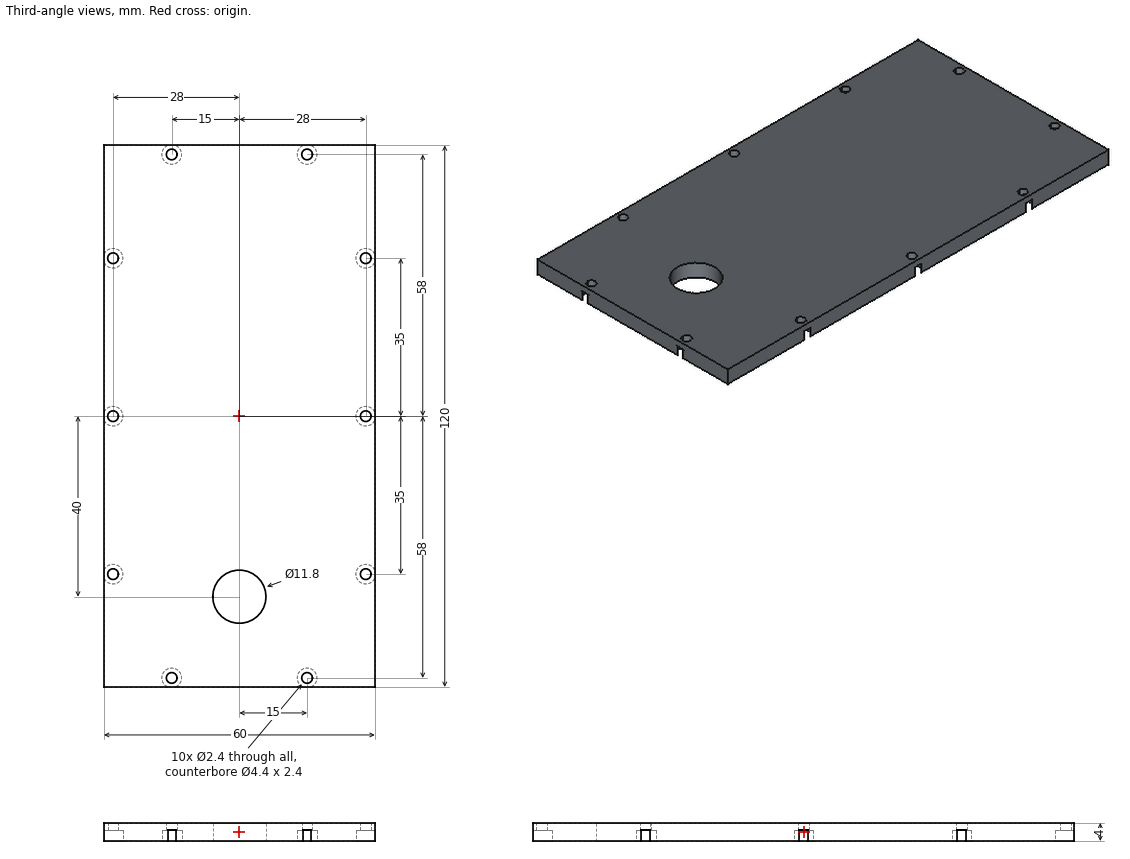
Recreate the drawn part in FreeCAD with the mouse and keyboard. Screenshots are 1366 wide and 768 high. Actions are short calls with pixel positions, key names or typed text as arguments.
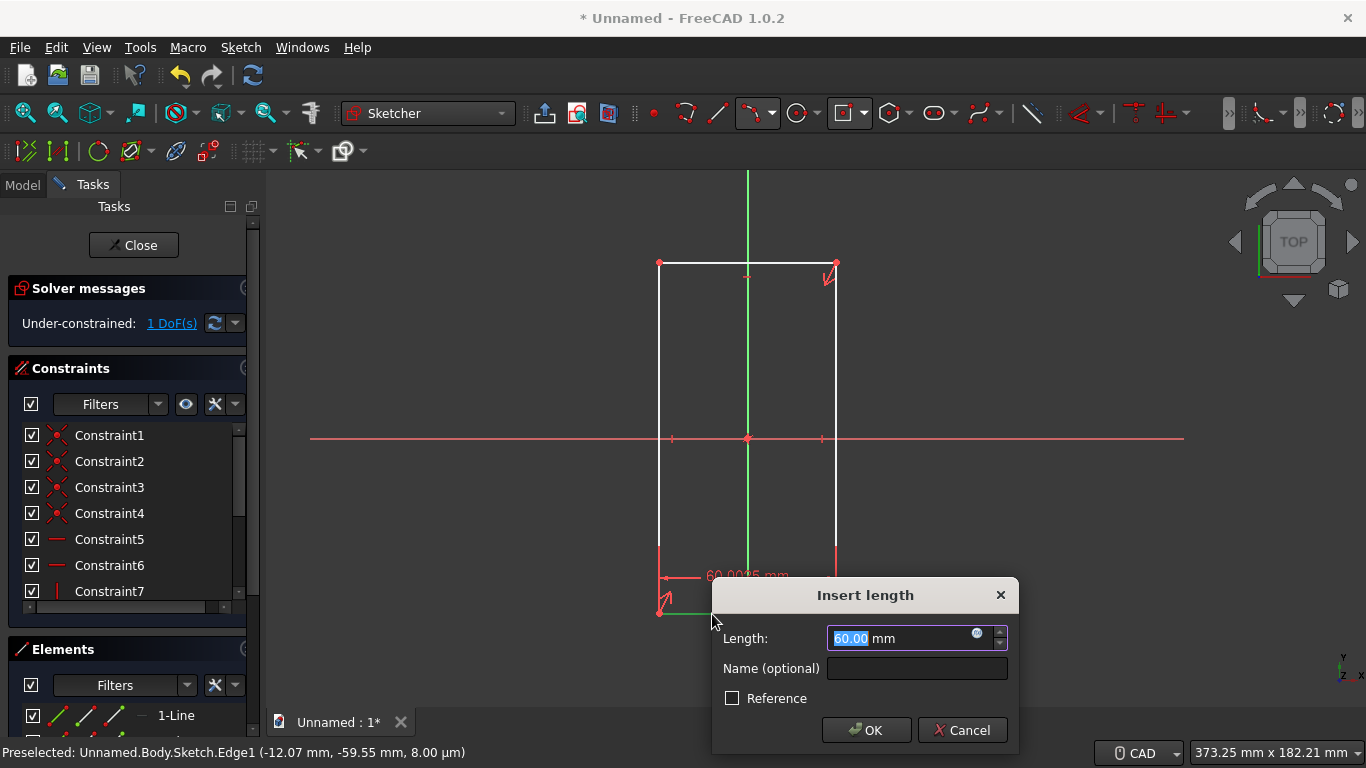
text(60)
key(Return)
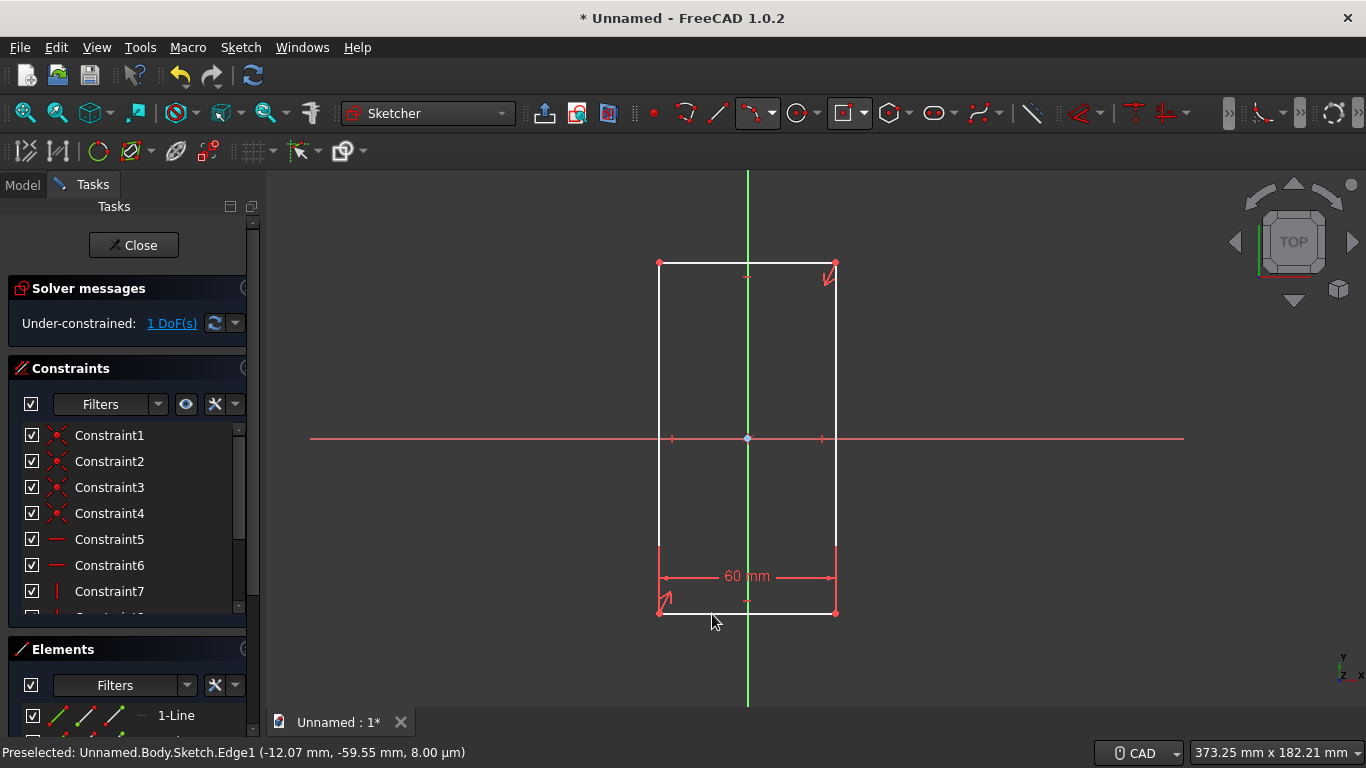
click(836, 509)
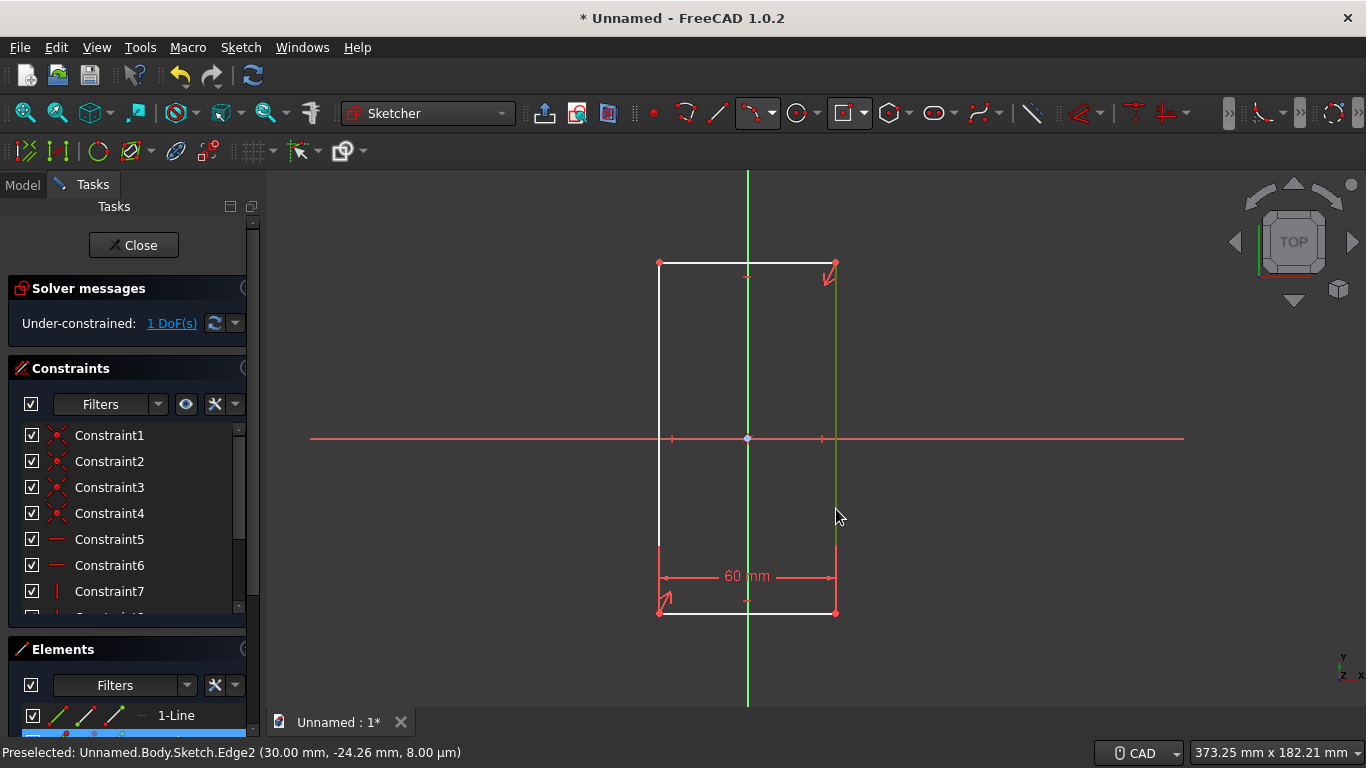
click(1102, 114)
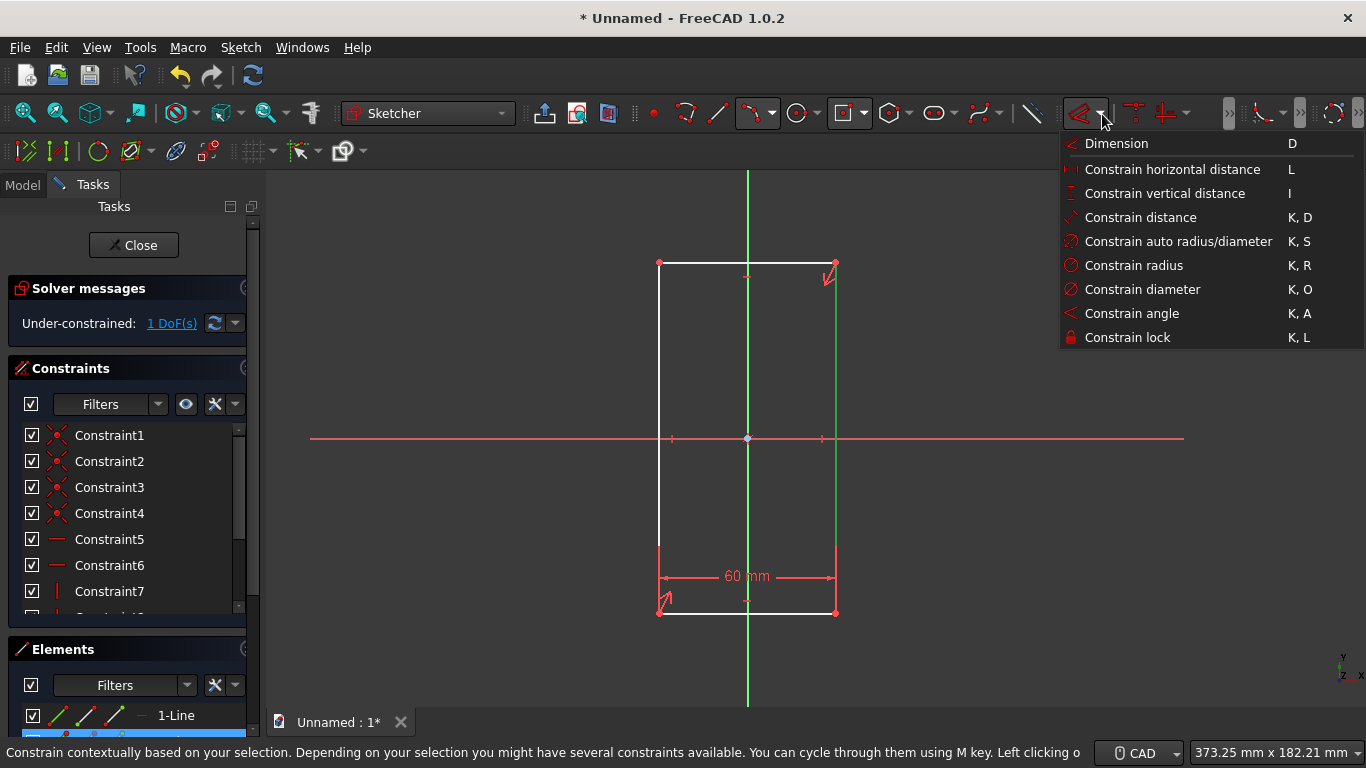
click(1212, 193)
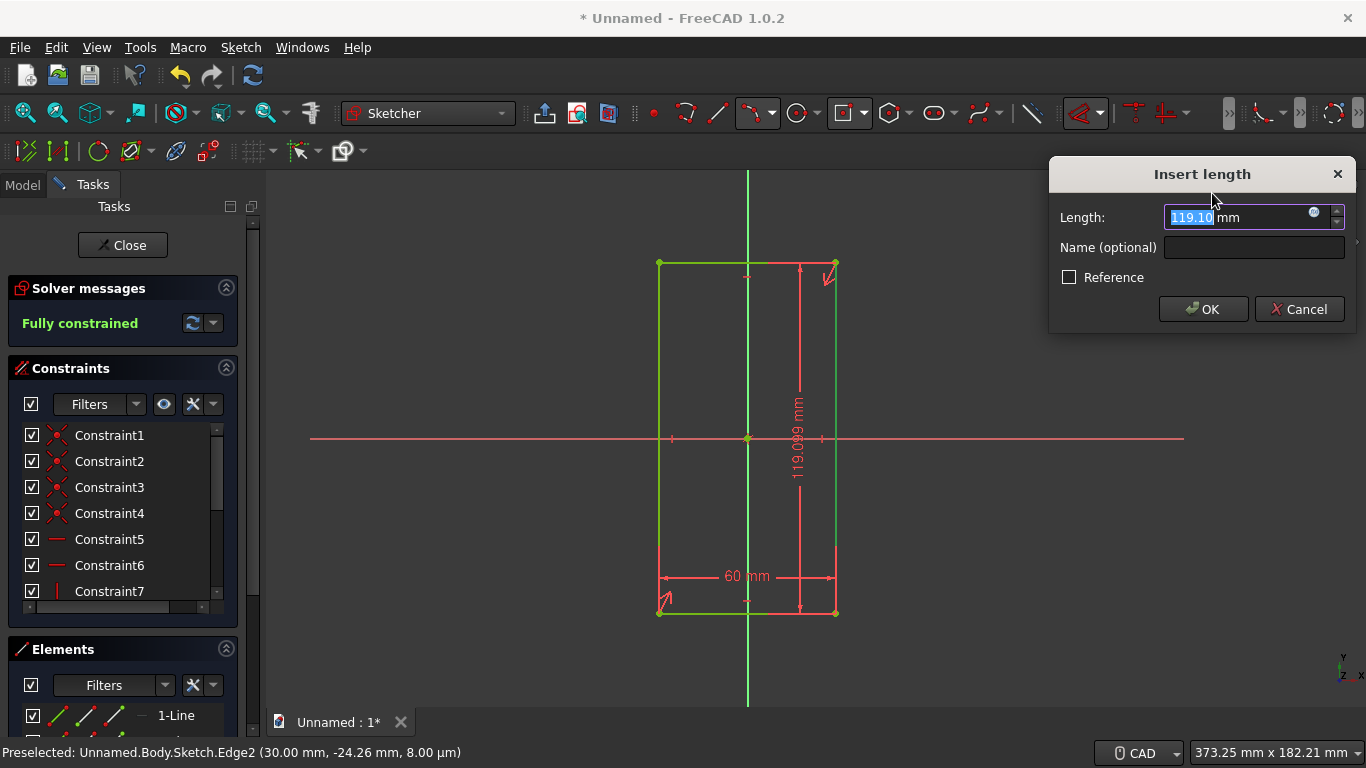
text(120)
key(Return)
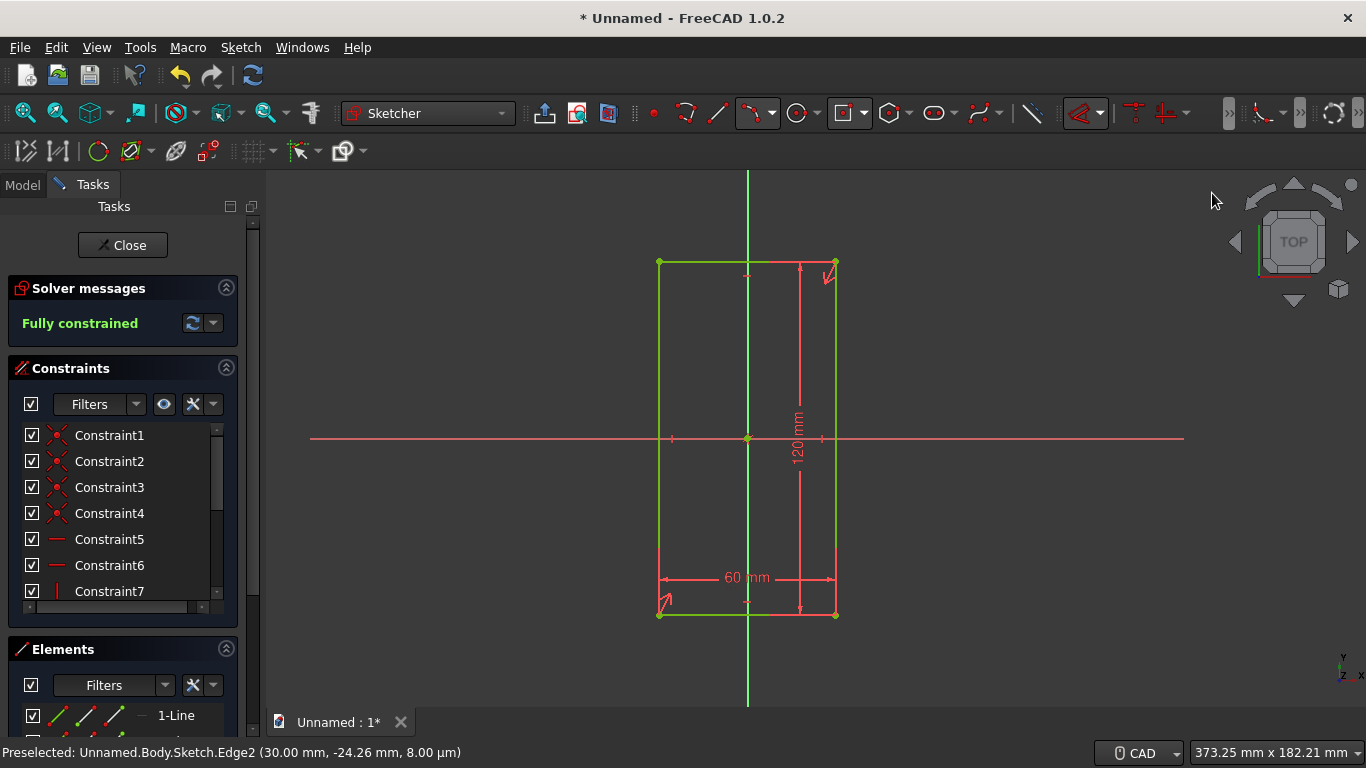
click(123, 245)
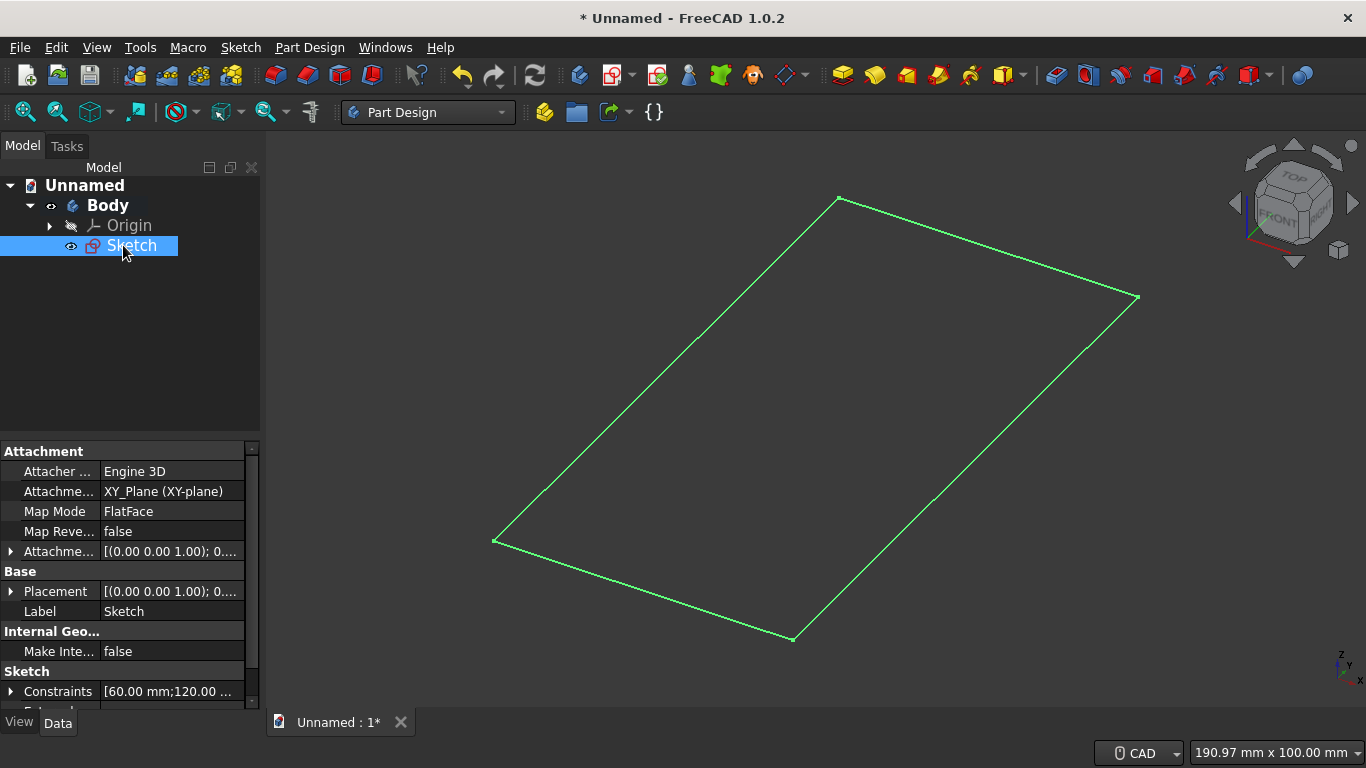
click(844, 76)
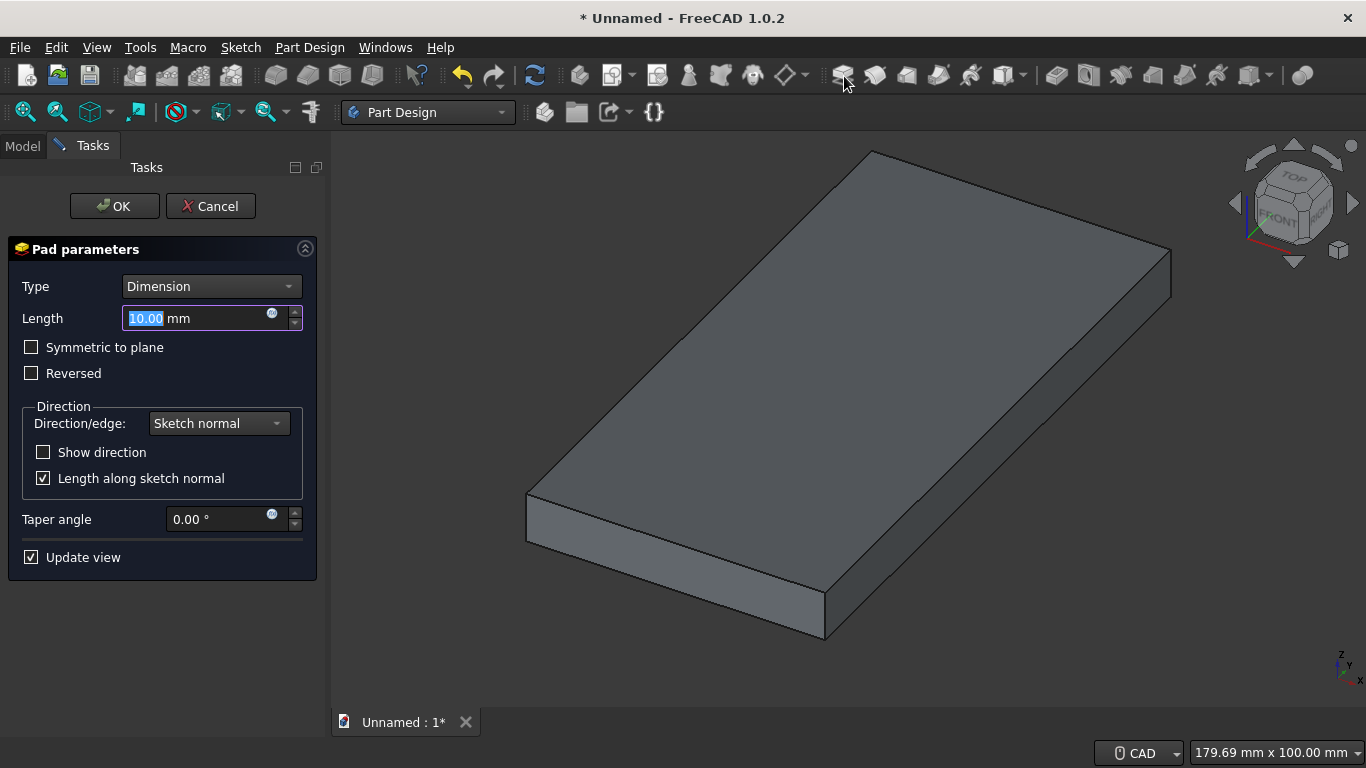
text(4)
key(Tab)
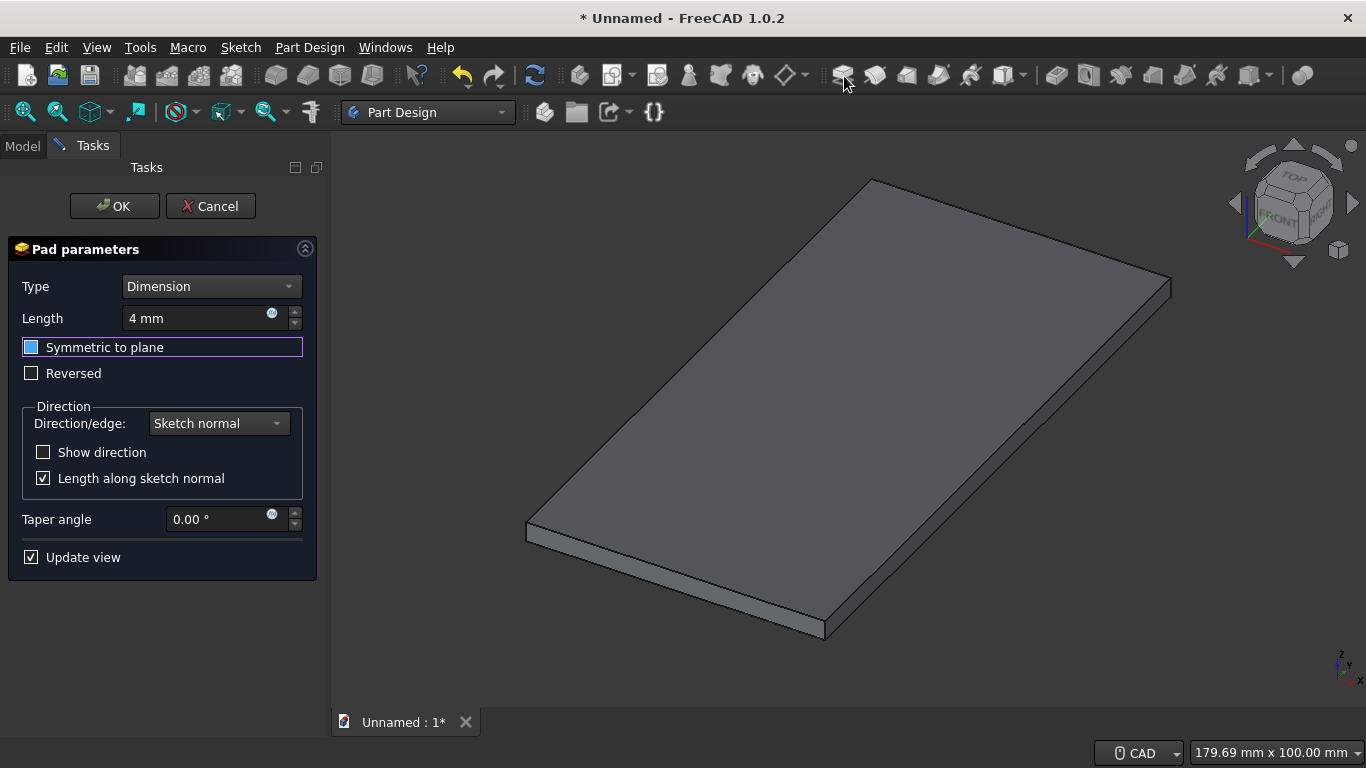
click(30, 347)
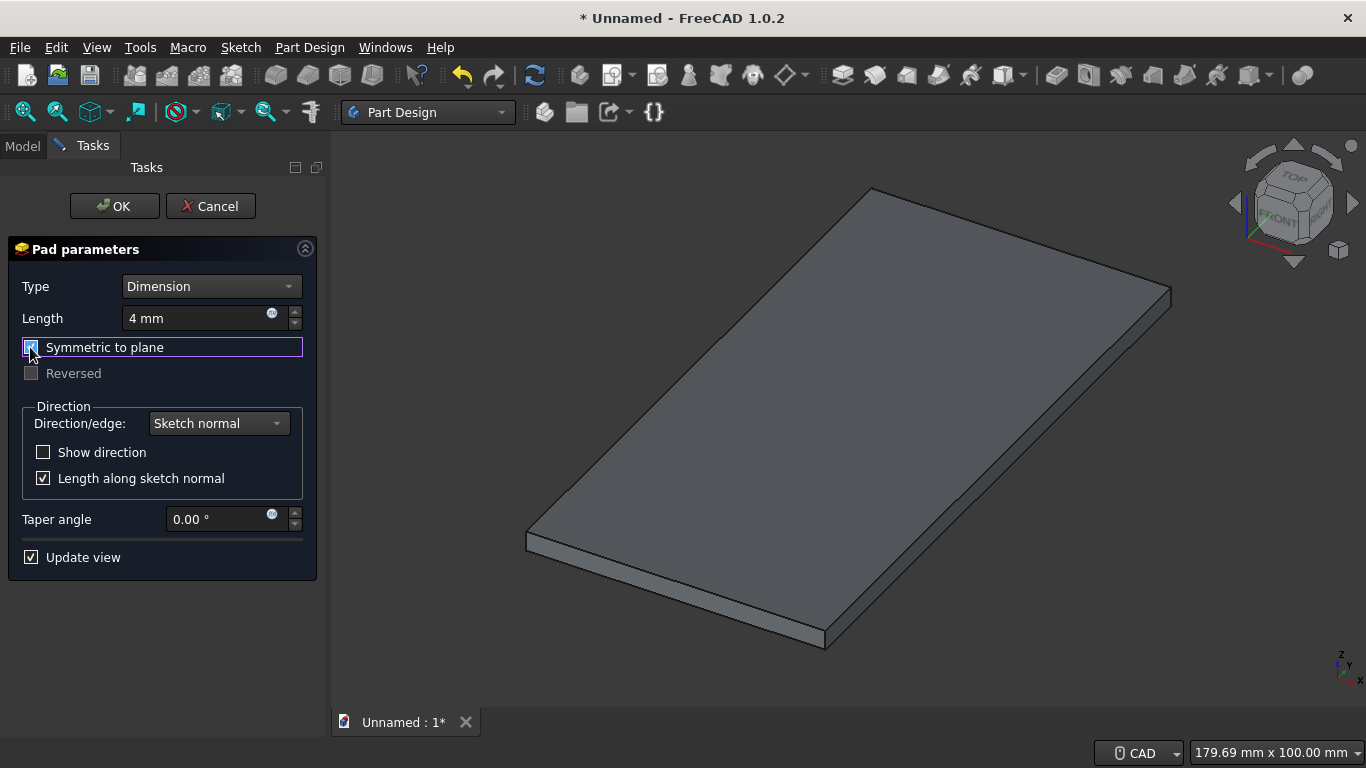
click(115, 206)